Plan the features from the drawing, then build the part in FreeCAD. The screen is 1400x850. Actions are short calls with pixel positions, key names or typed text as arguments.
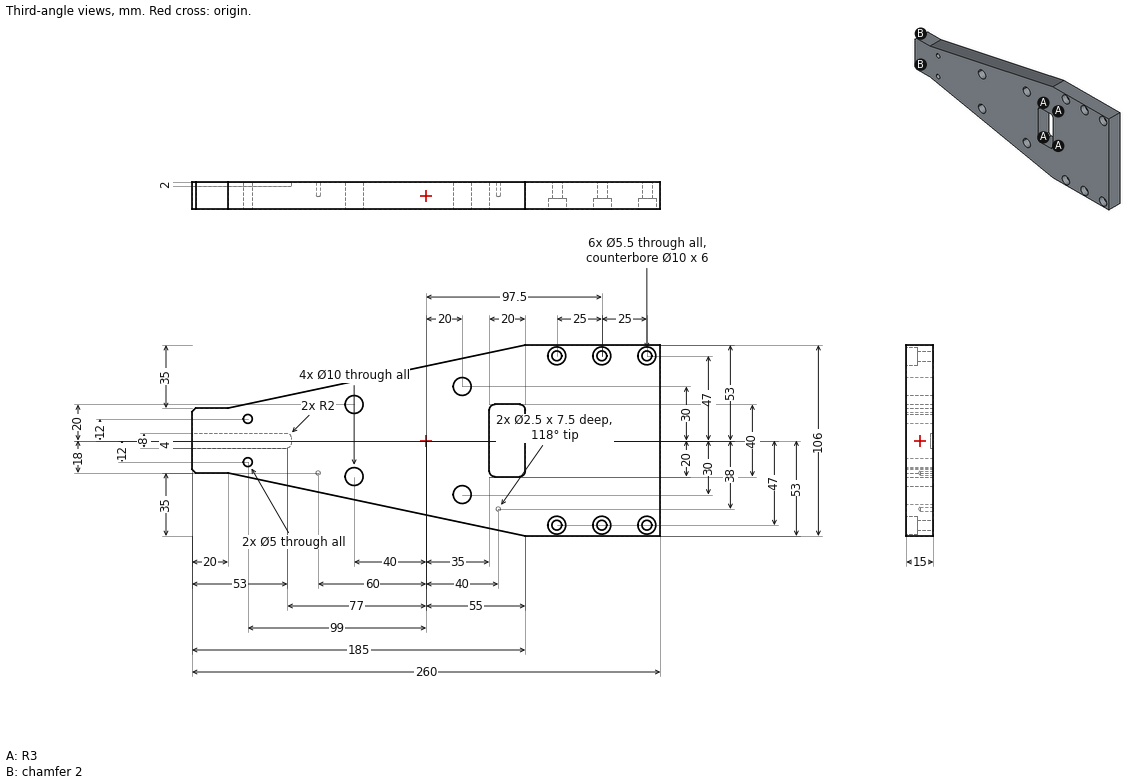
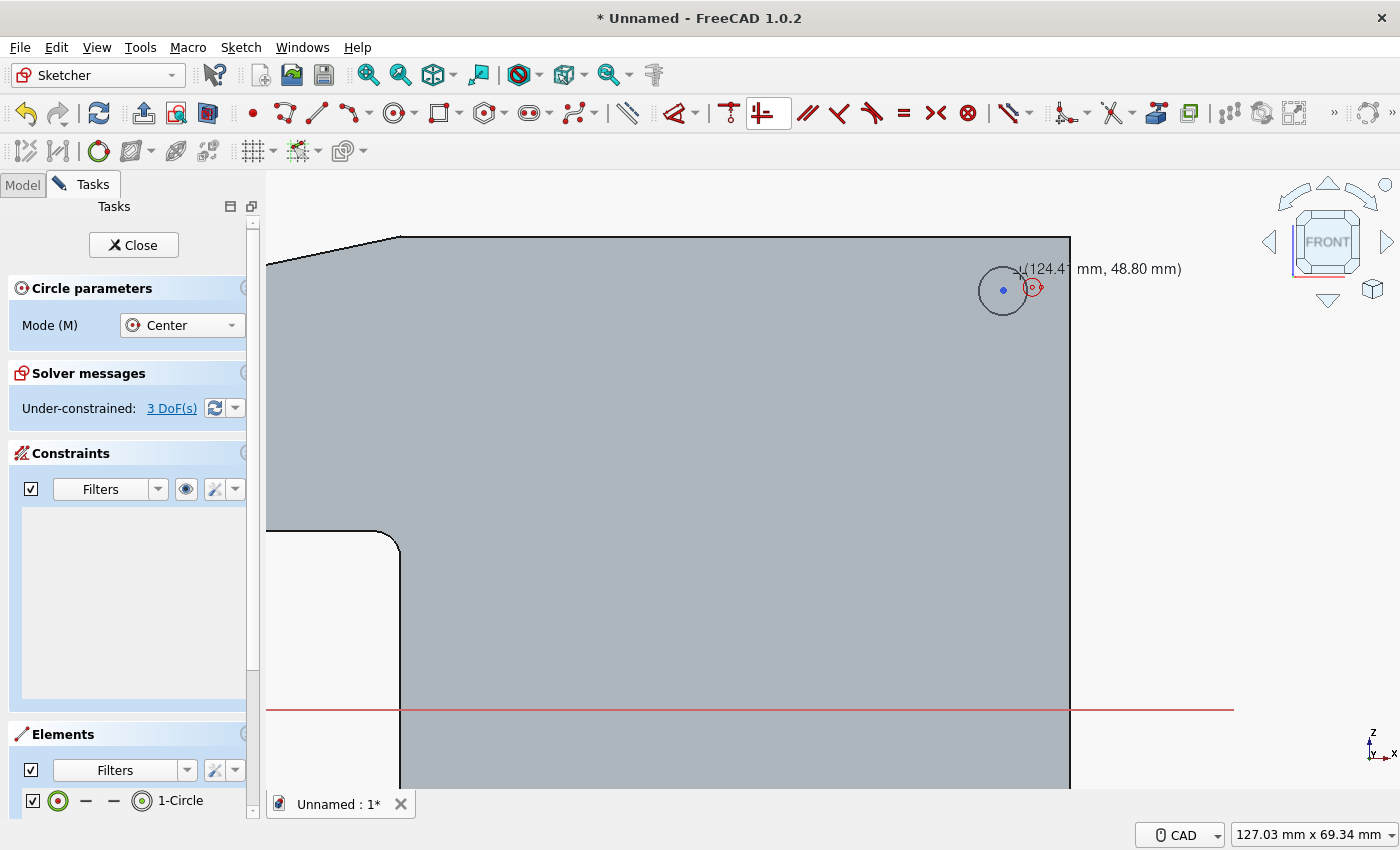
click(780, 290)
click(797, 273)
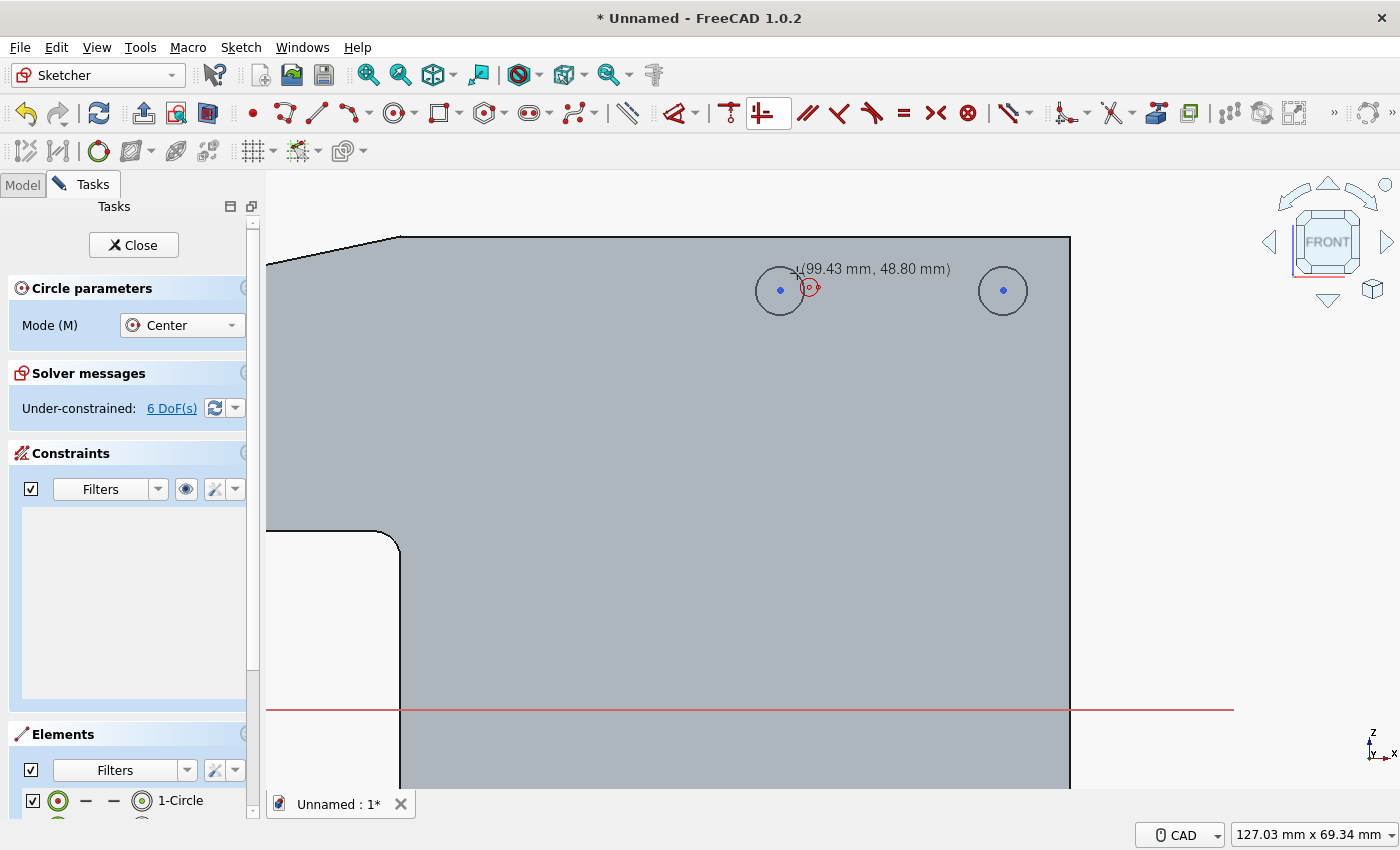
click(557, 290)
click(574, 273)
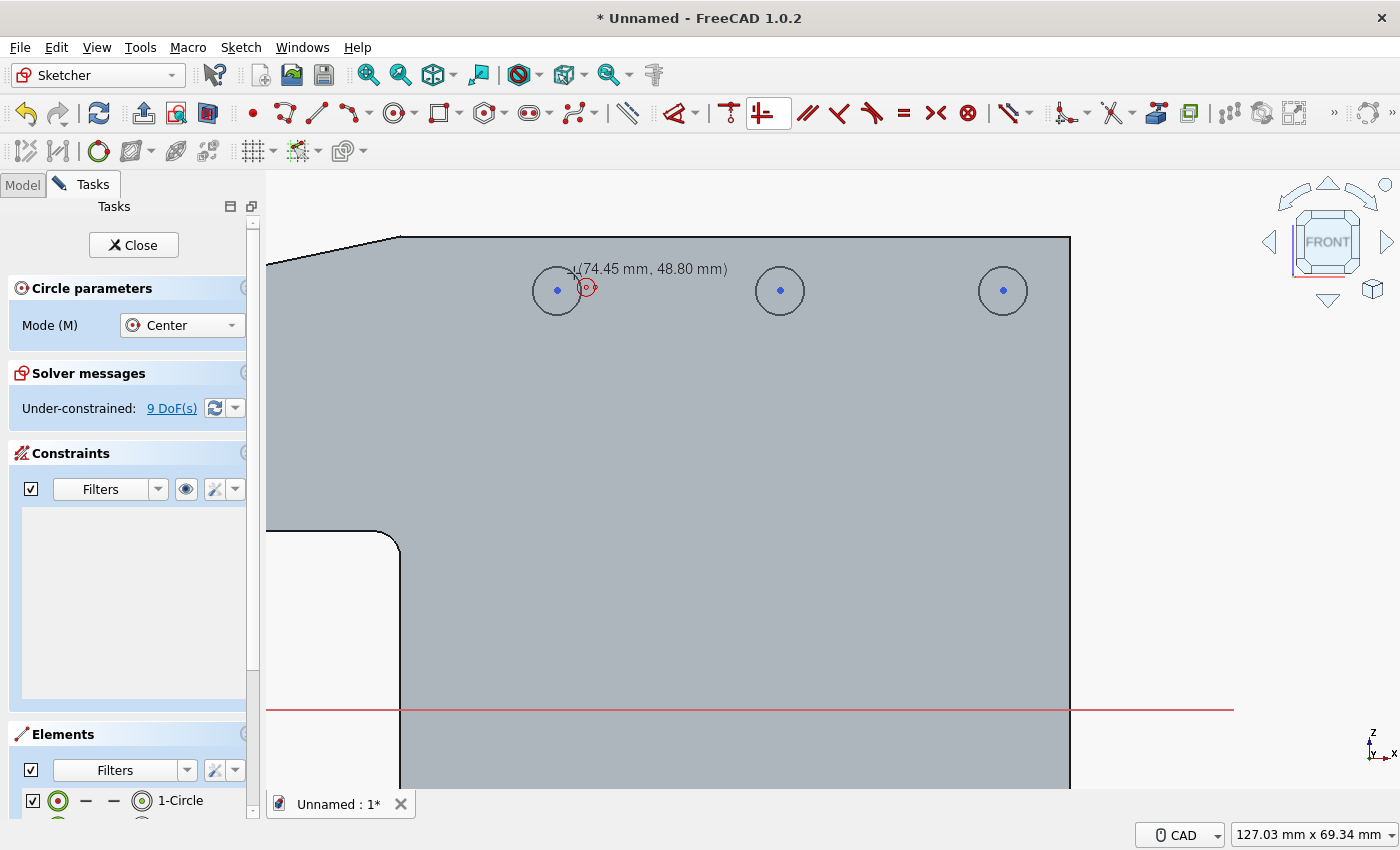
scroll(1006, 292, down, 4)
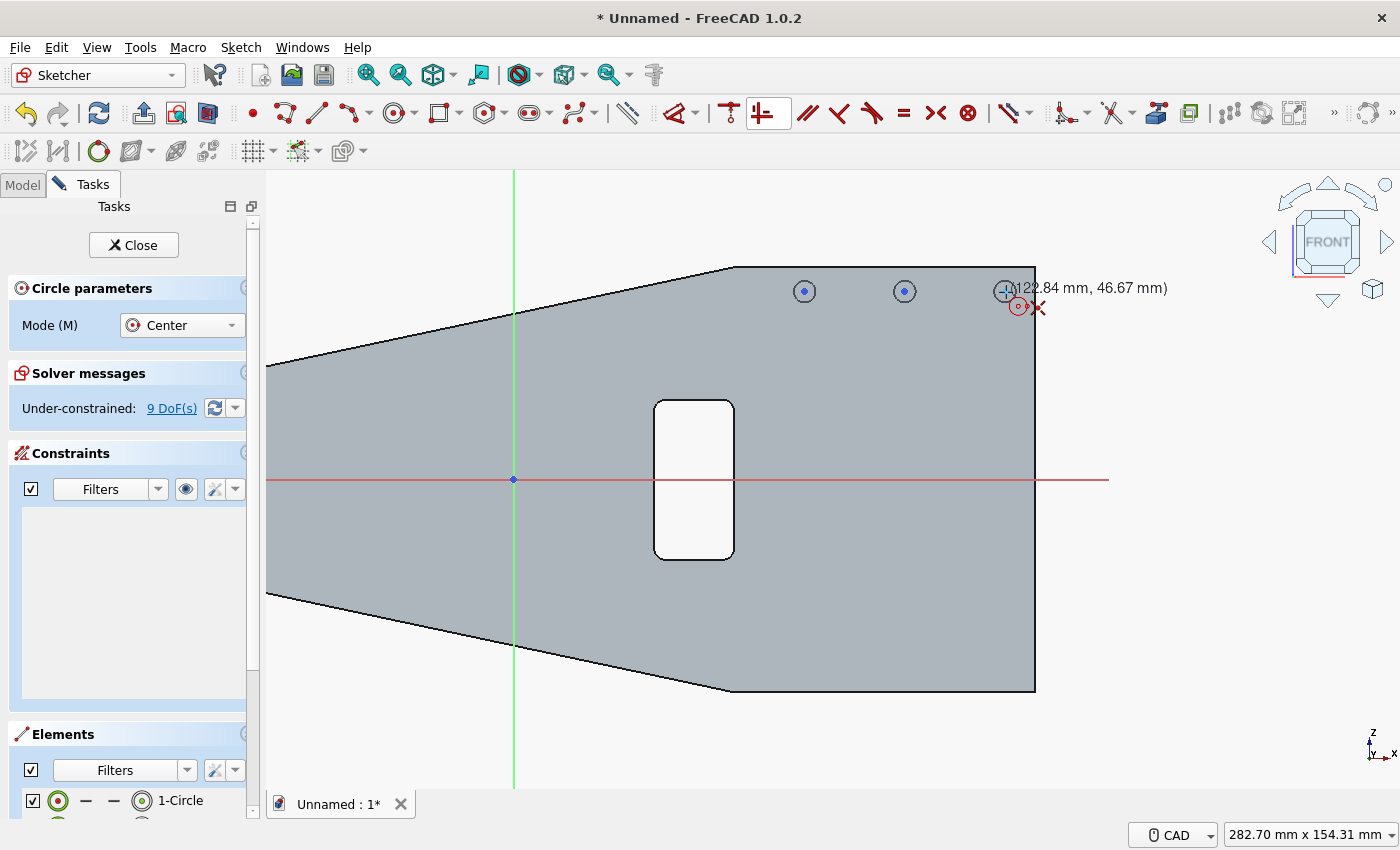
scroll(804, 668, up, 4)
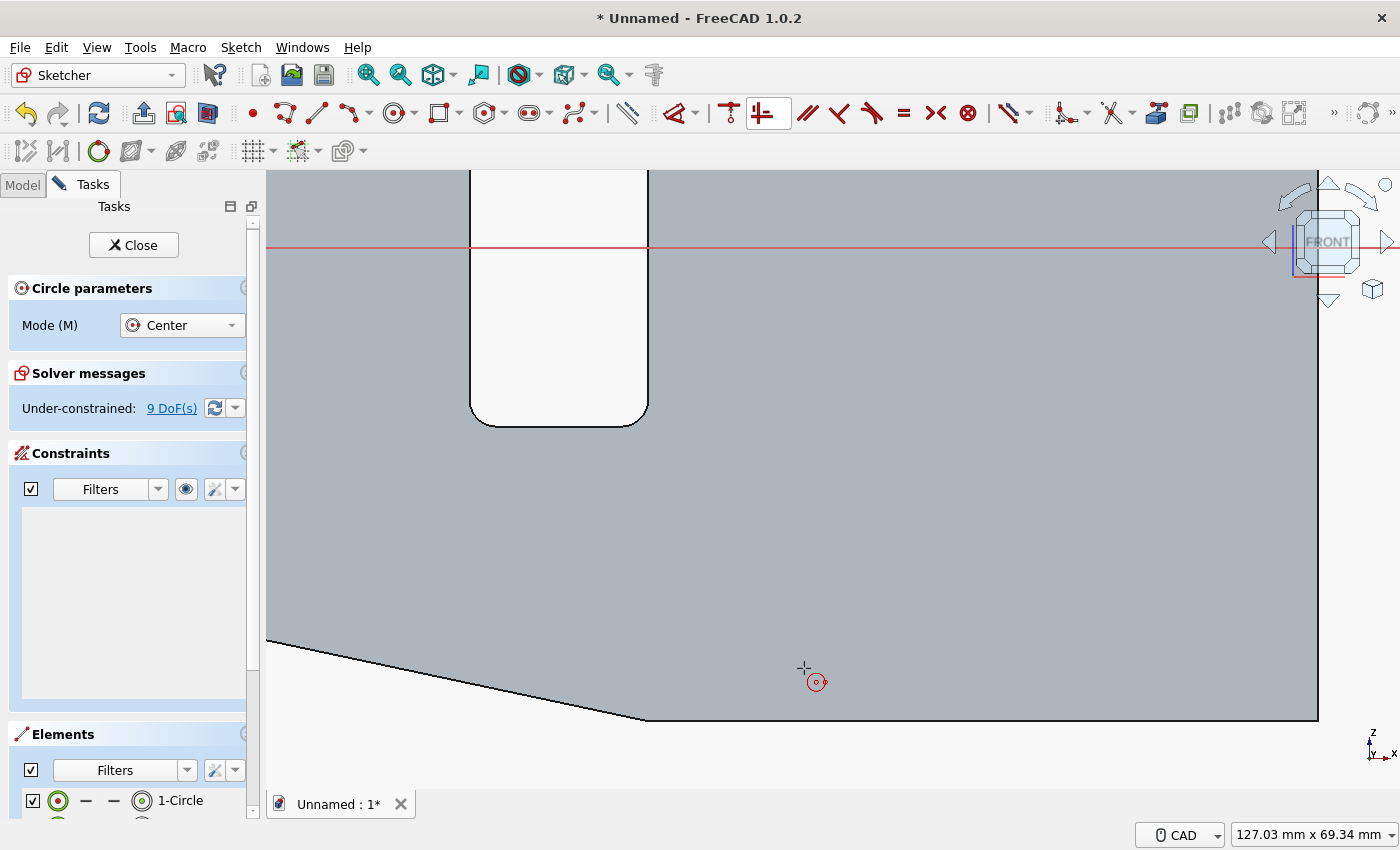
click(804, 668)
click(822, 650)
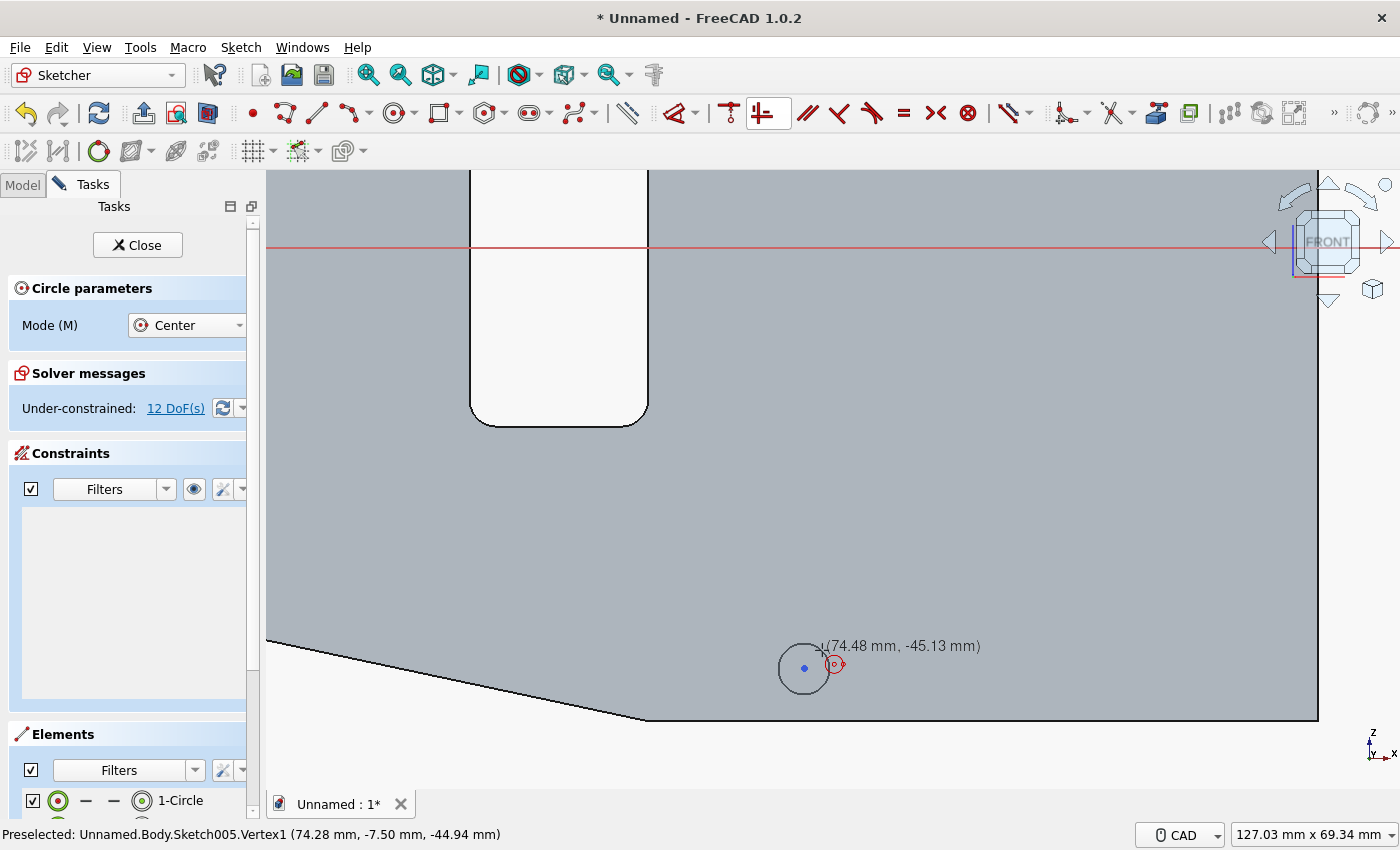
click(1028, 668)
click(1045, 650)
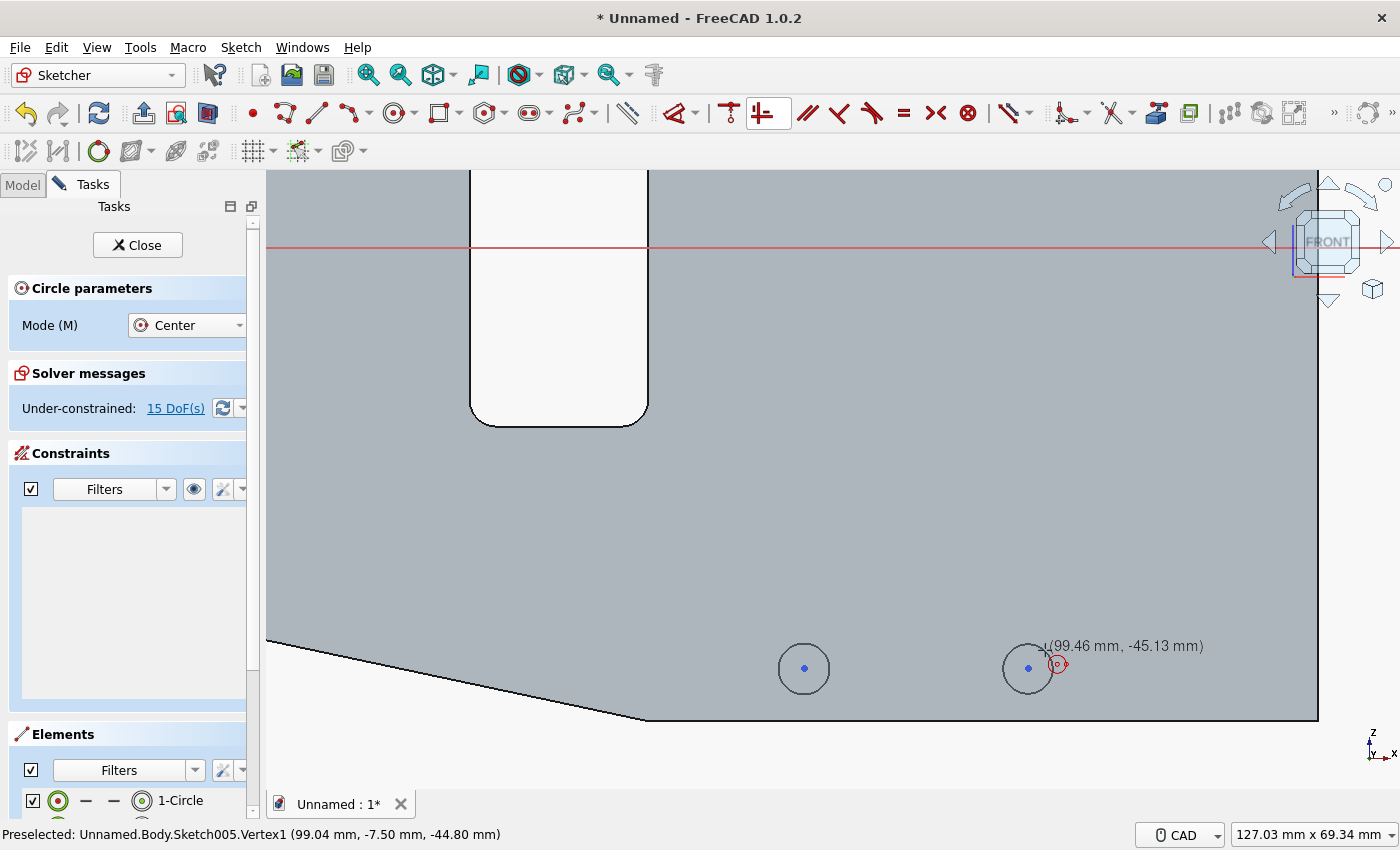
scroll(804, 668, down, 4)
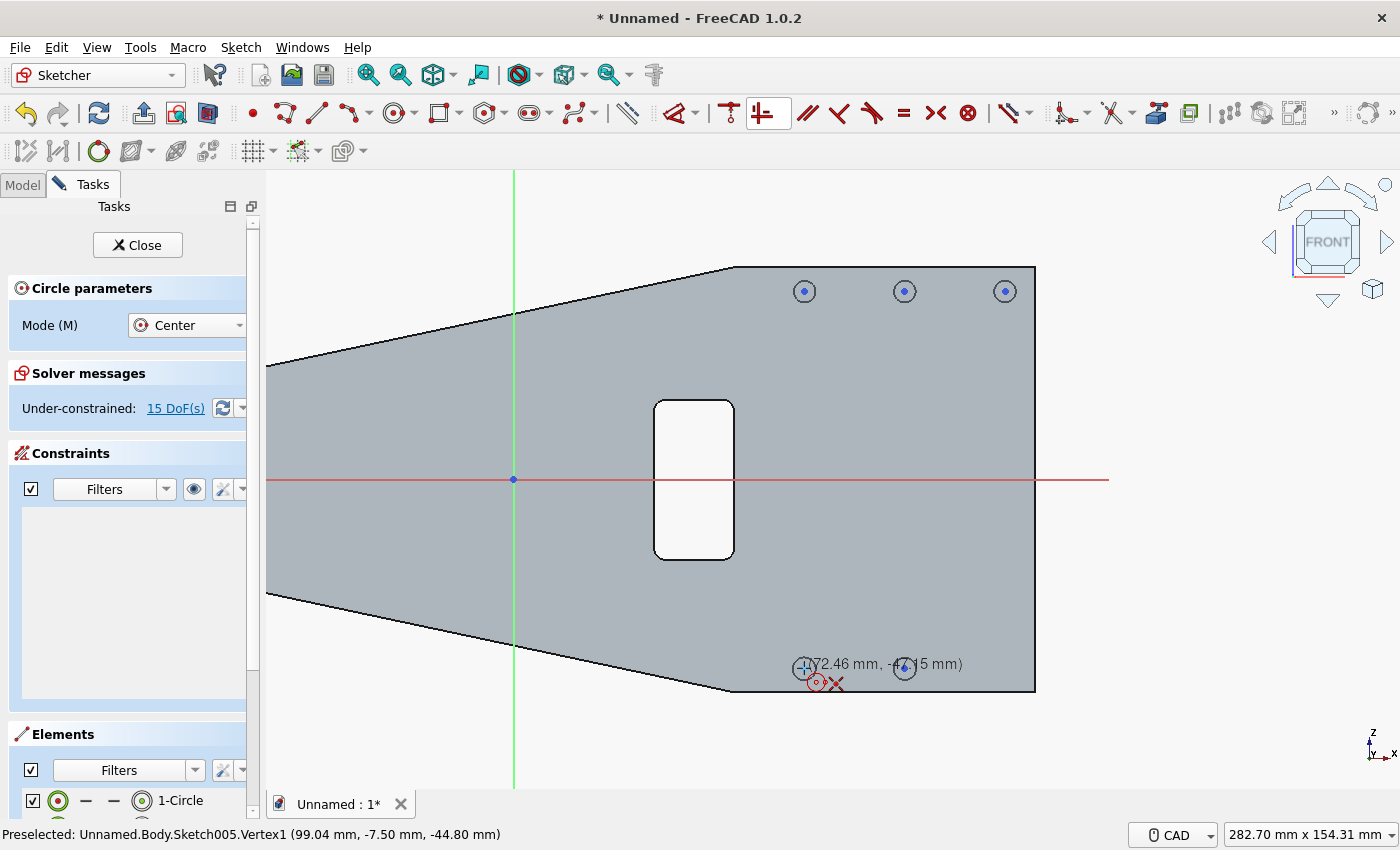
scroll(1005, 668, up, 4)